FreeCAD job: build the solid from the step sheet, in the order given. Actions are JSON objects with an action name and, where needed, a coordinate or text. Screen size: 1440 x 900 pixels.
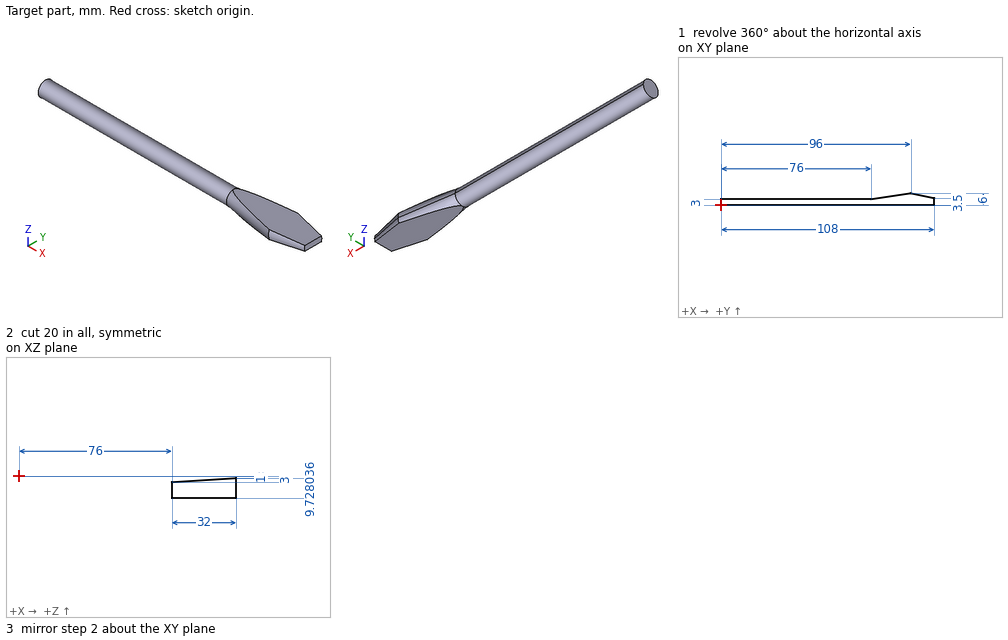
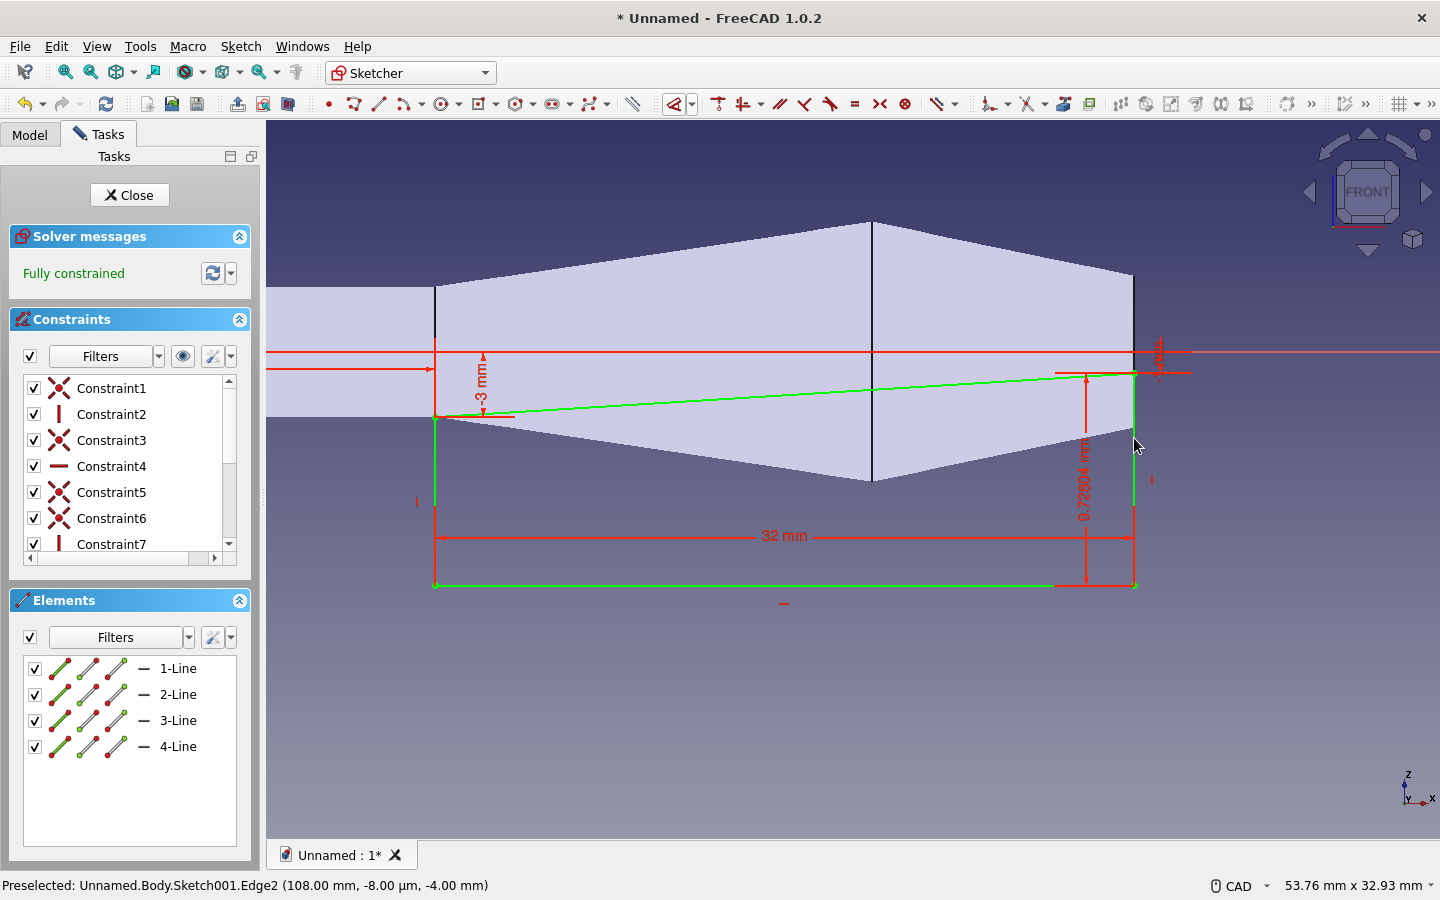
{"action": "left_click", "coordinate": [130, 195]}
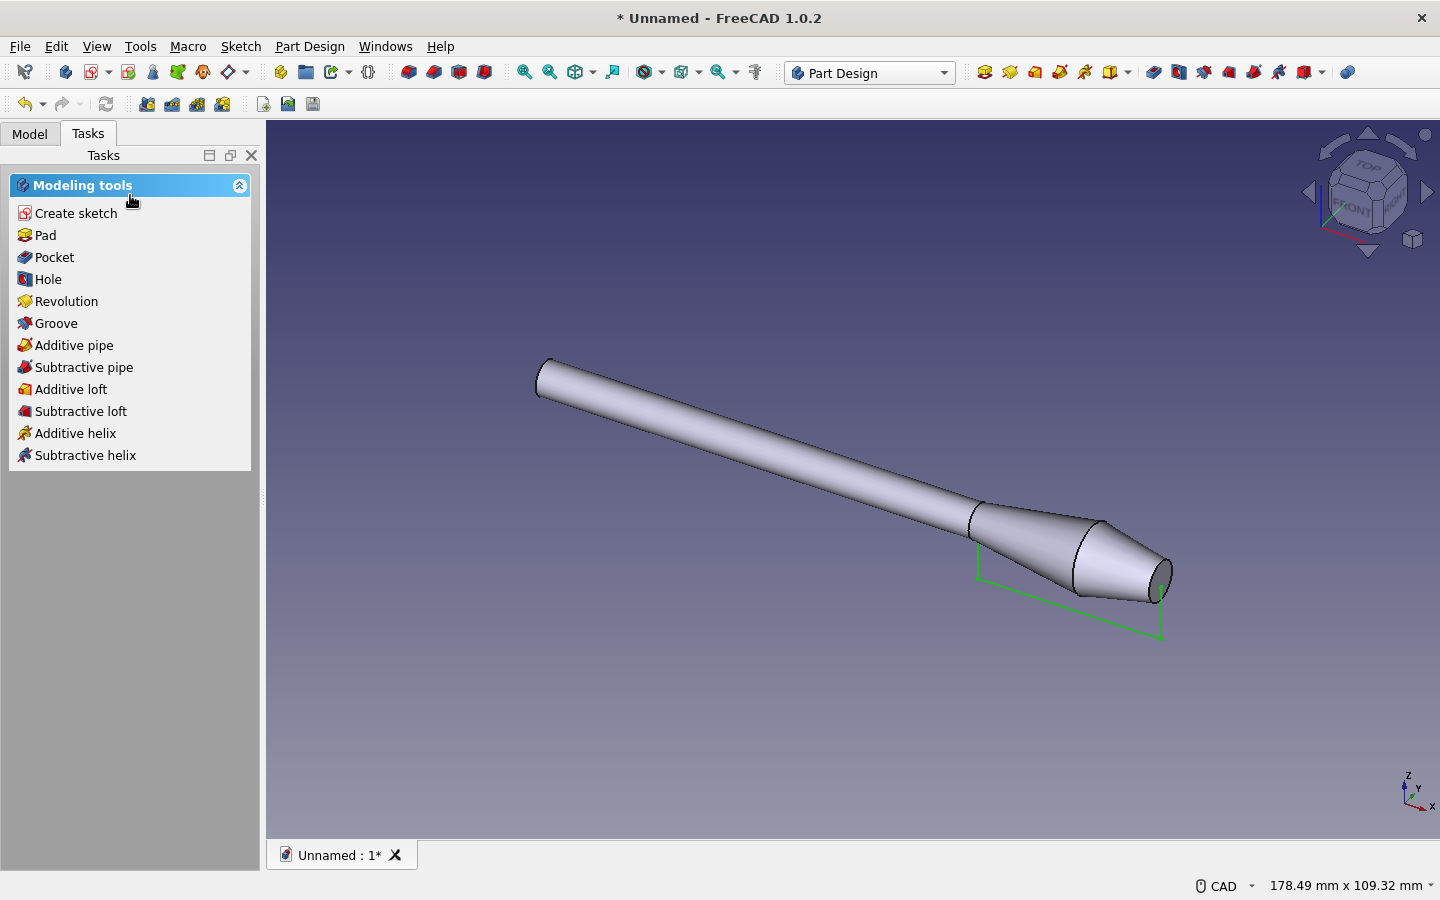
{"action": "left_click", "coordinate": [1154, 72]}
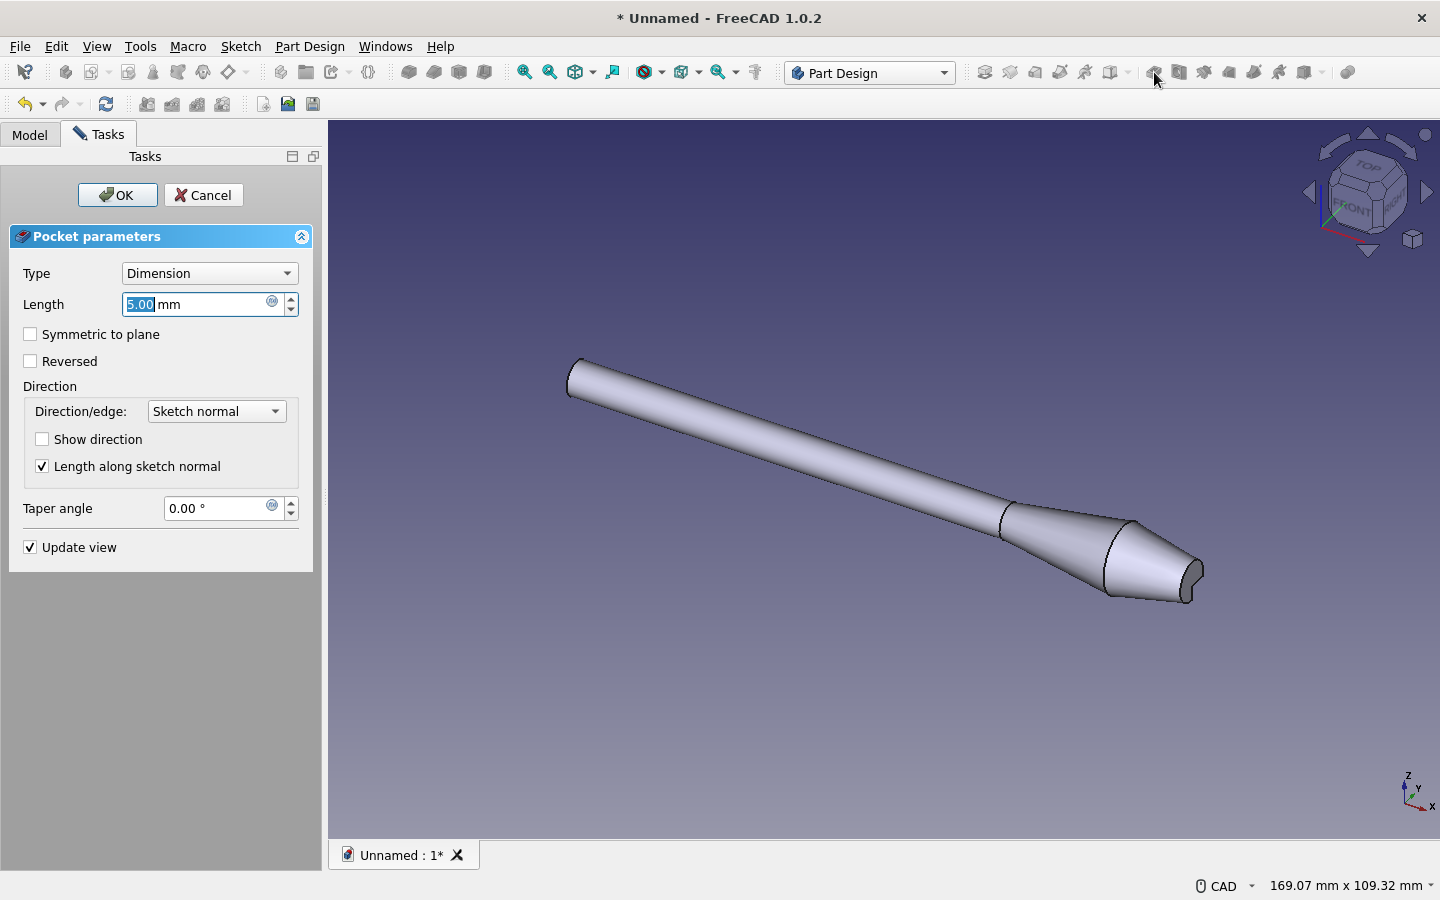
{"action": "type", "text": "20"}
{"action": "key", "text": "Tab"}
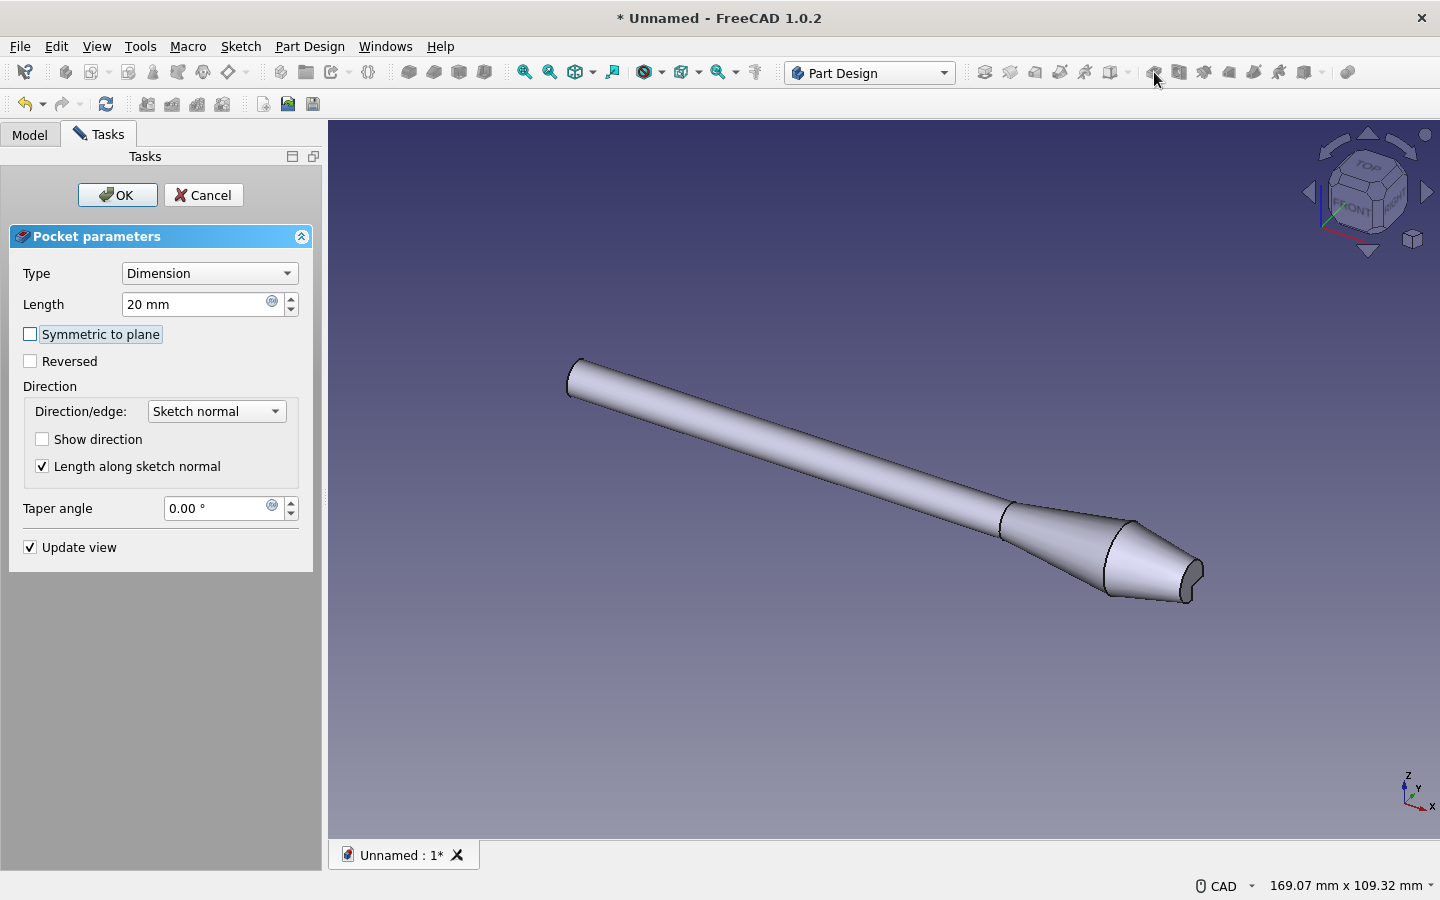
{"action": "left_click", "coordinate": [31, 334]}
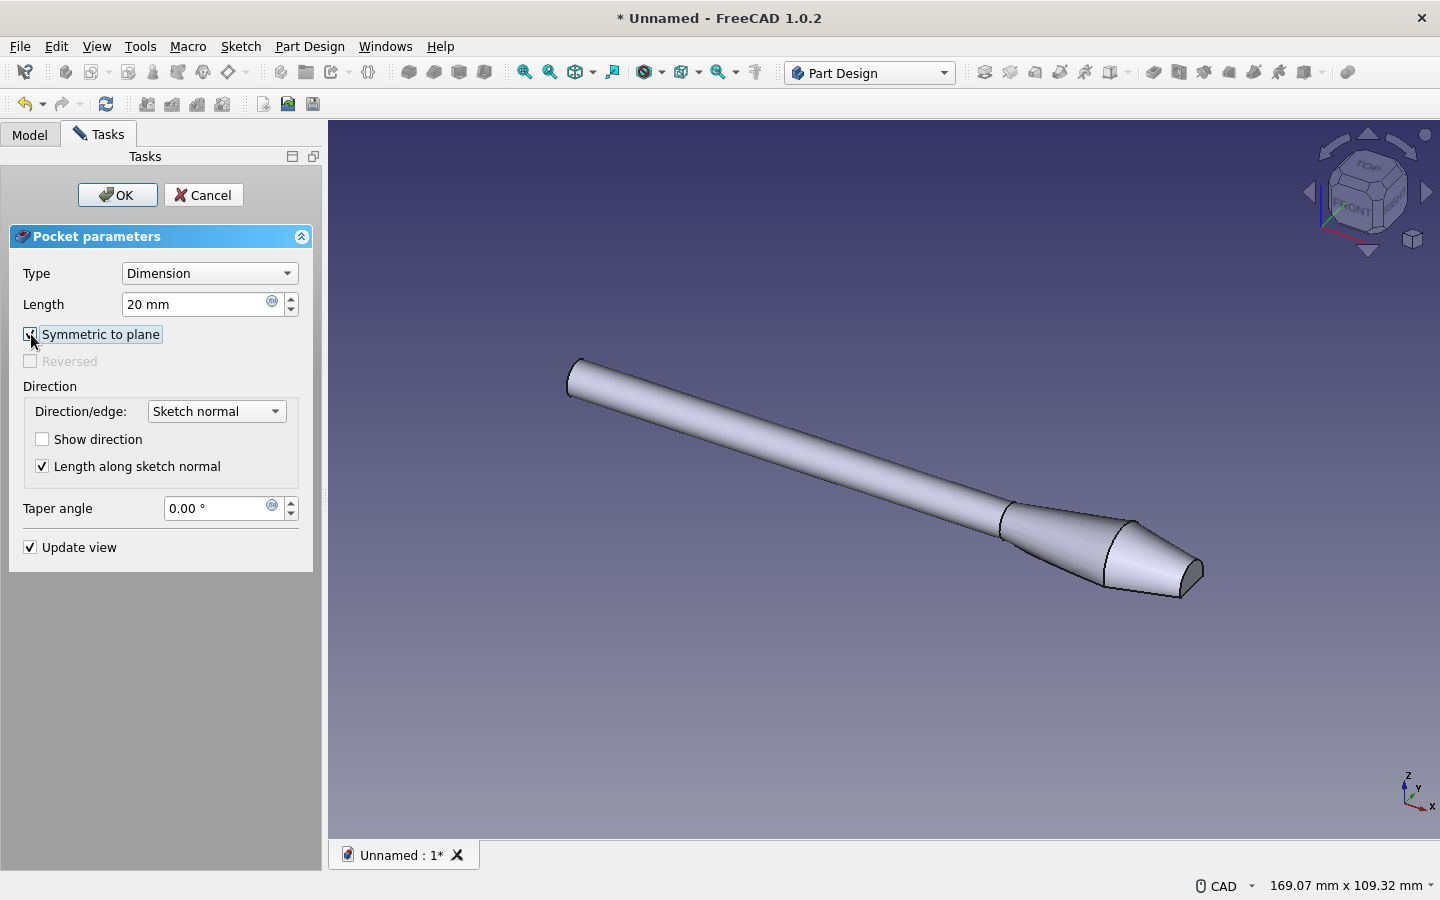
{"action": "left_click", "coordinate": [118, 195]}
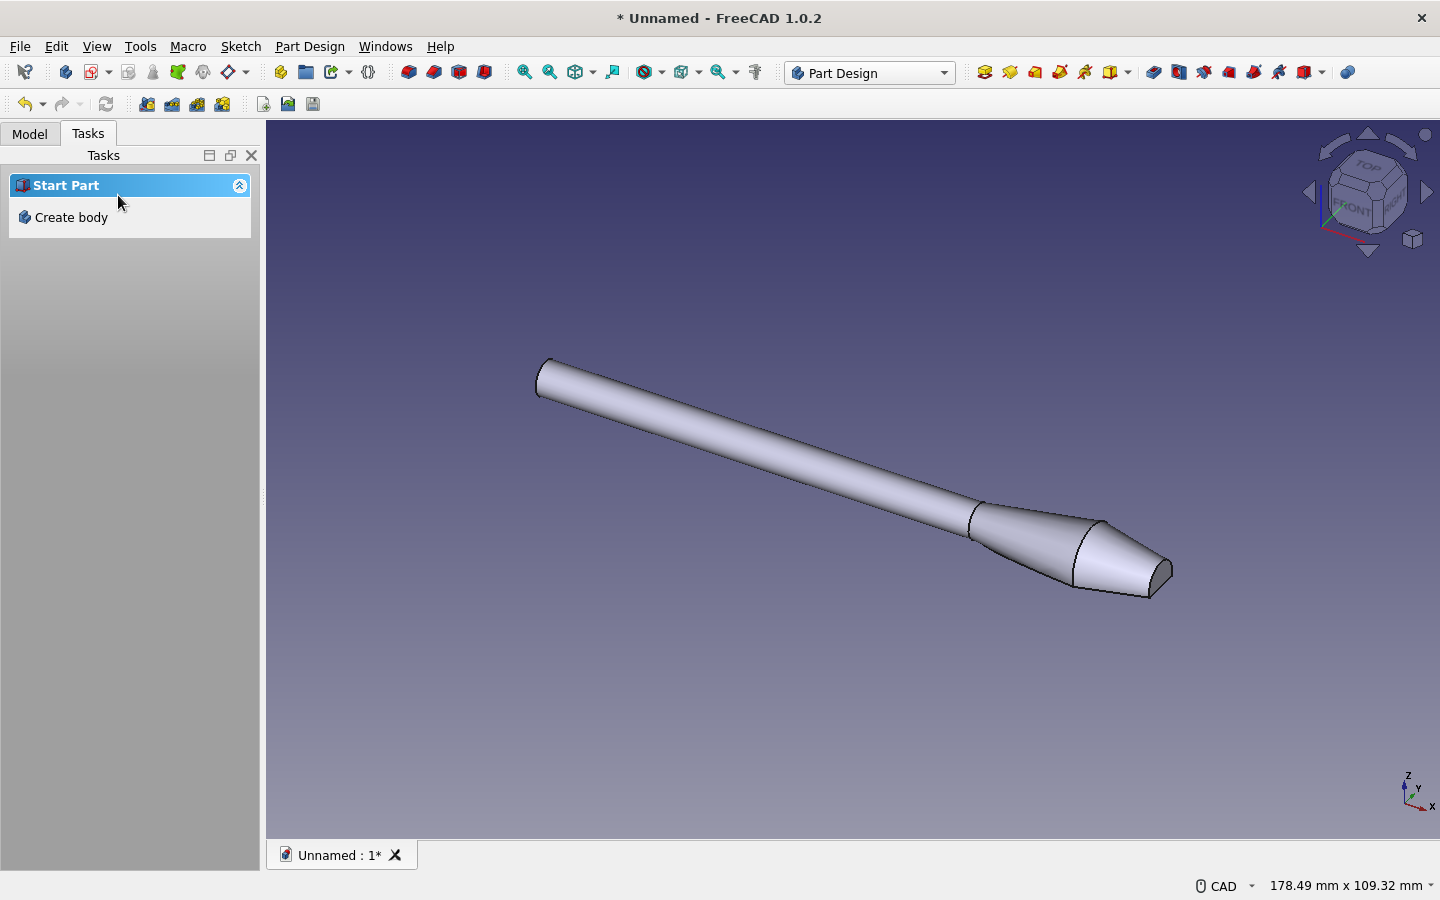
{"action": "left_click", "coordinate": [30, 134]}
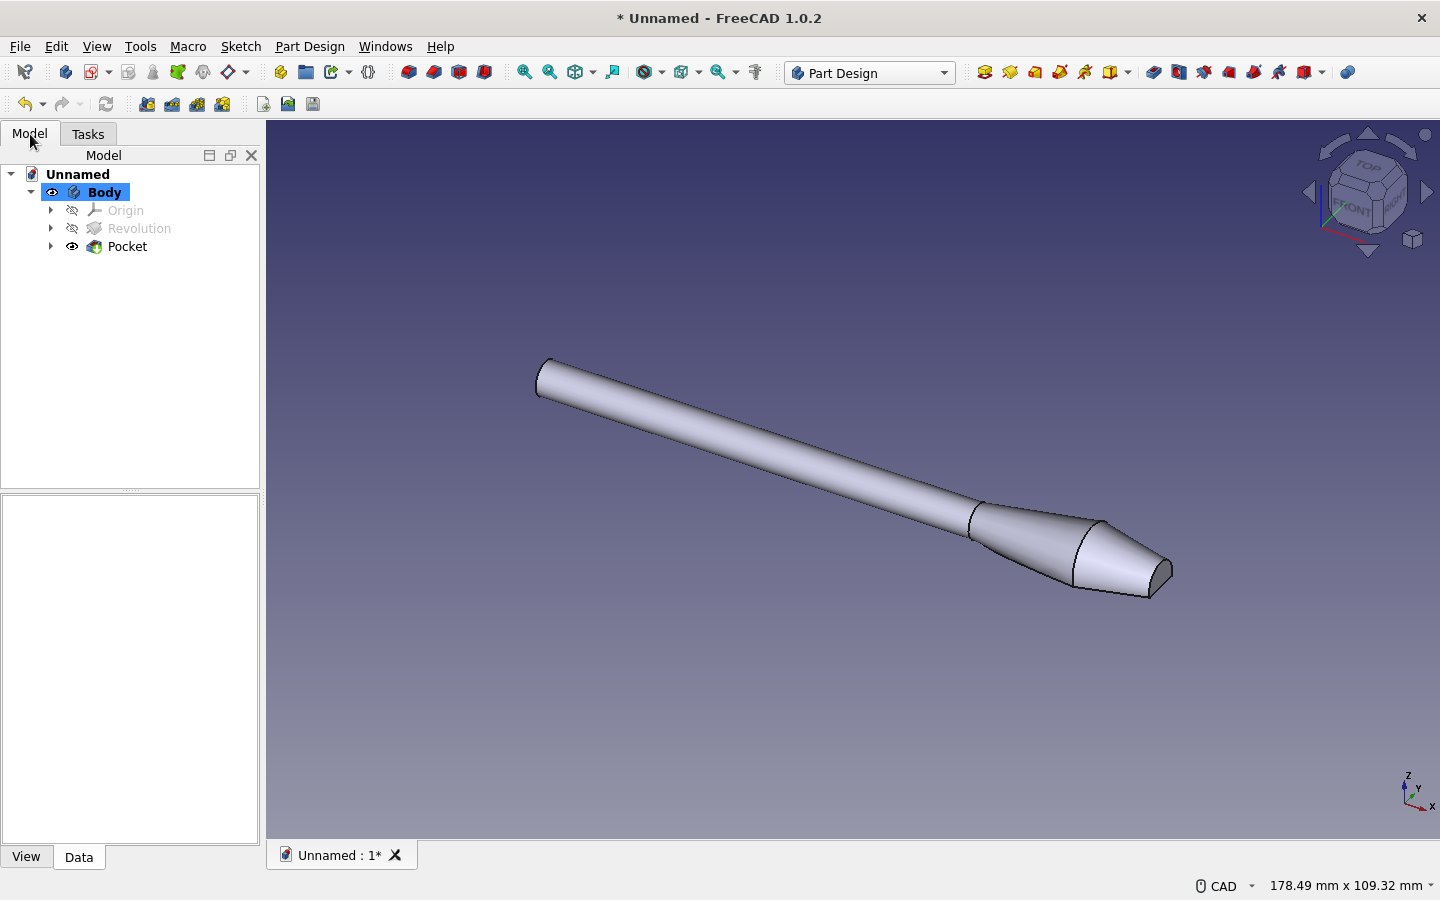
{"action": "left_click", "coordinate": [117, 246]}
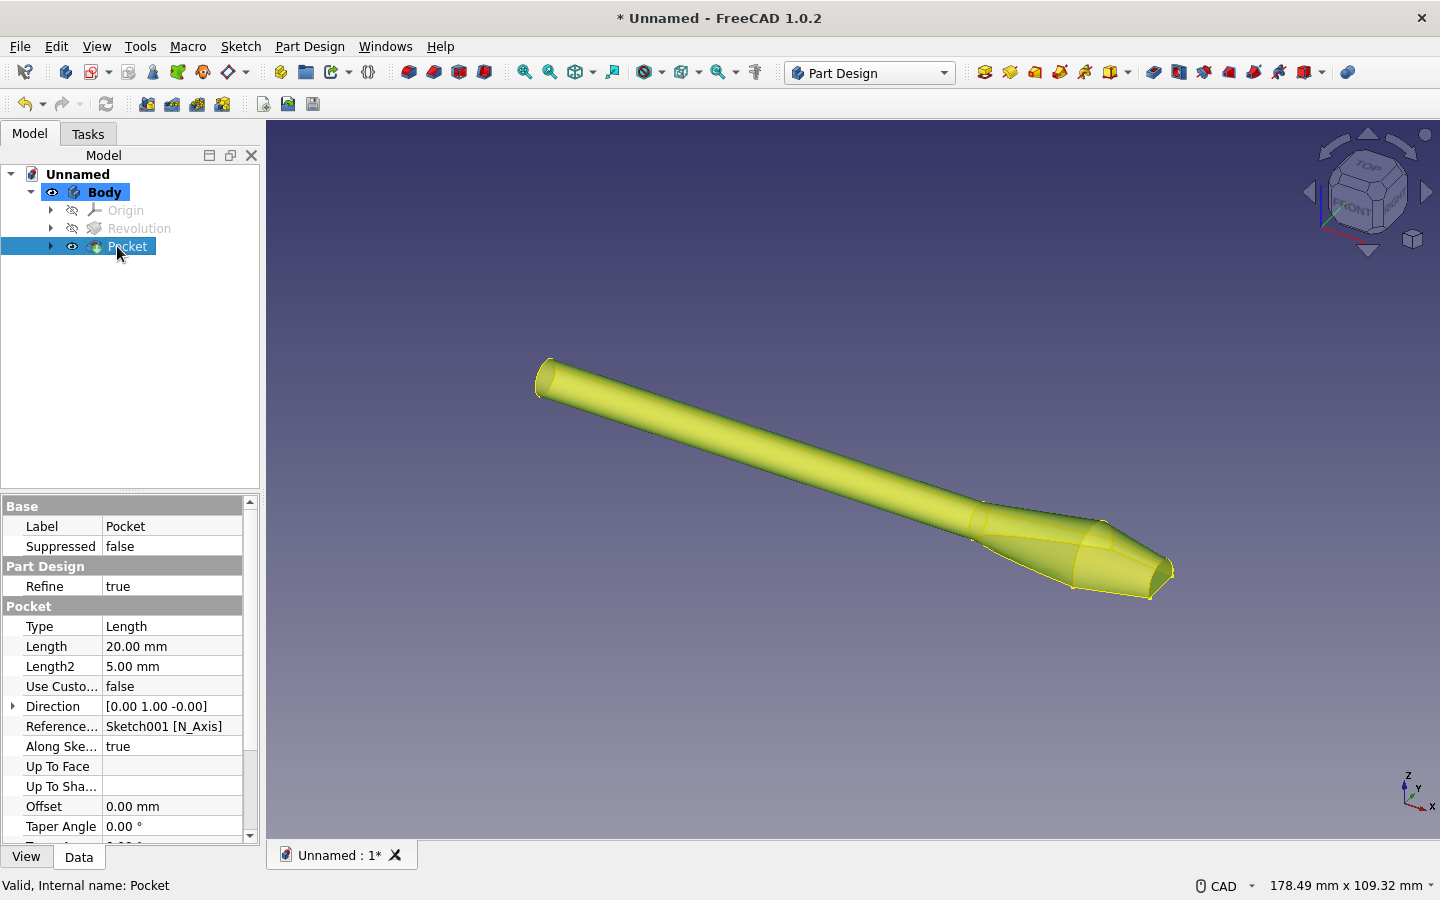
{"action": "left_click", "coordinate": [147, 104]}